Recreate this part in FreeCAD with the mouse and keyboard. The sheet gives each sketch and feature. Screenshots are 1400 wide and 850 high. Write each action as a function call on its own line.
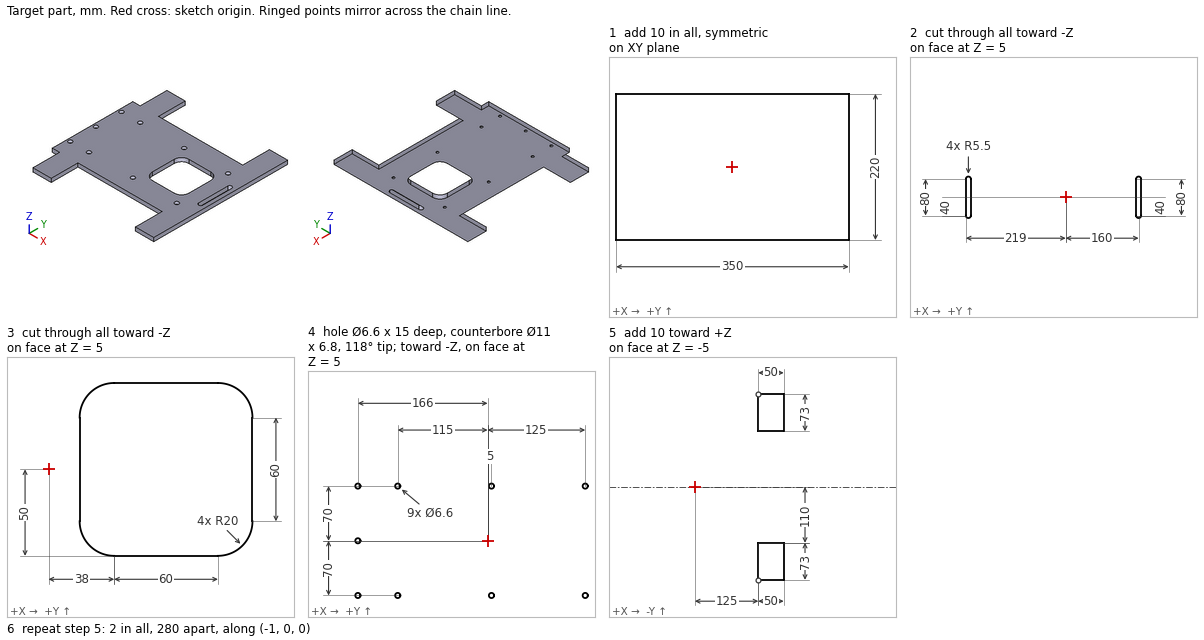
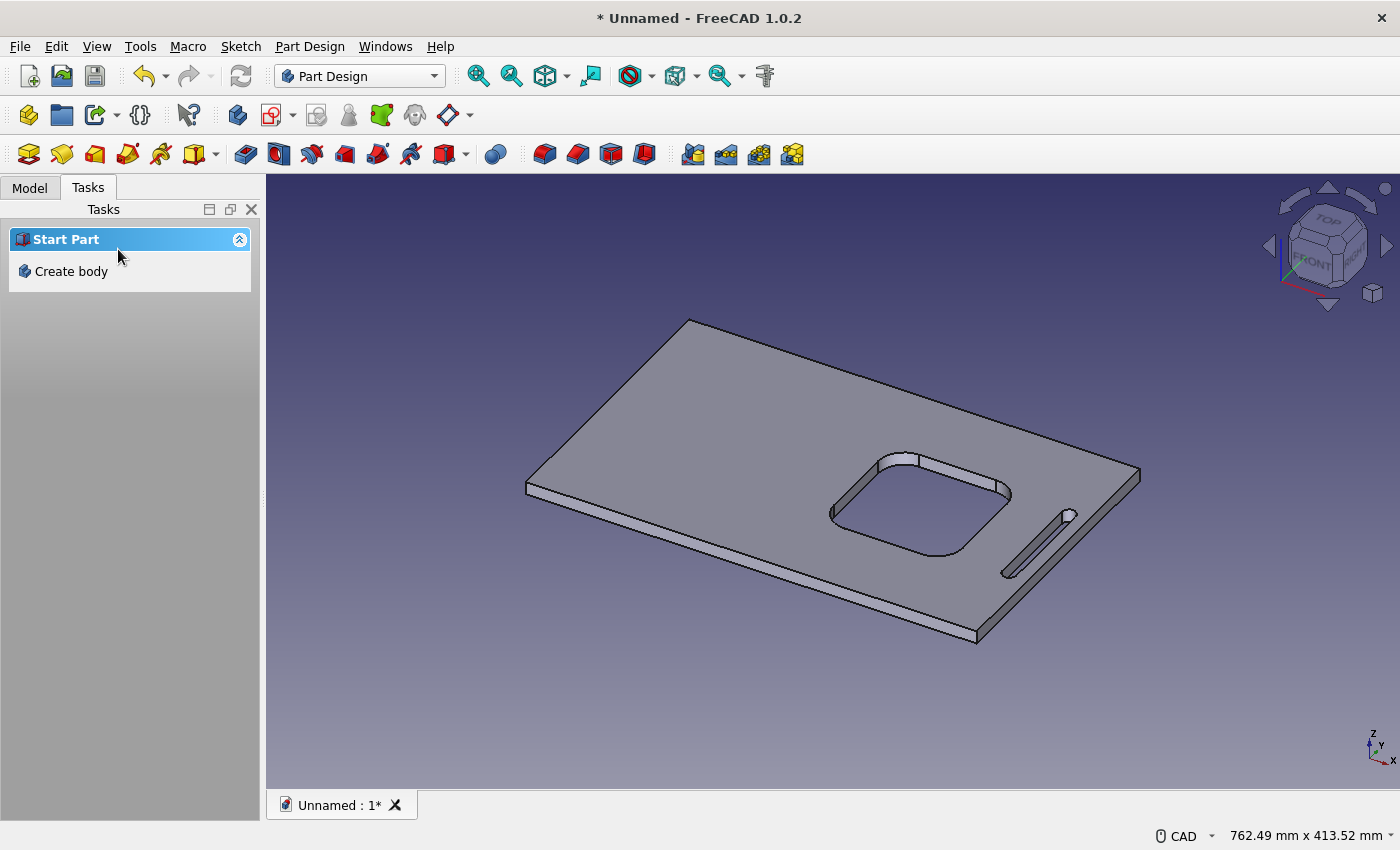
click(728, 409)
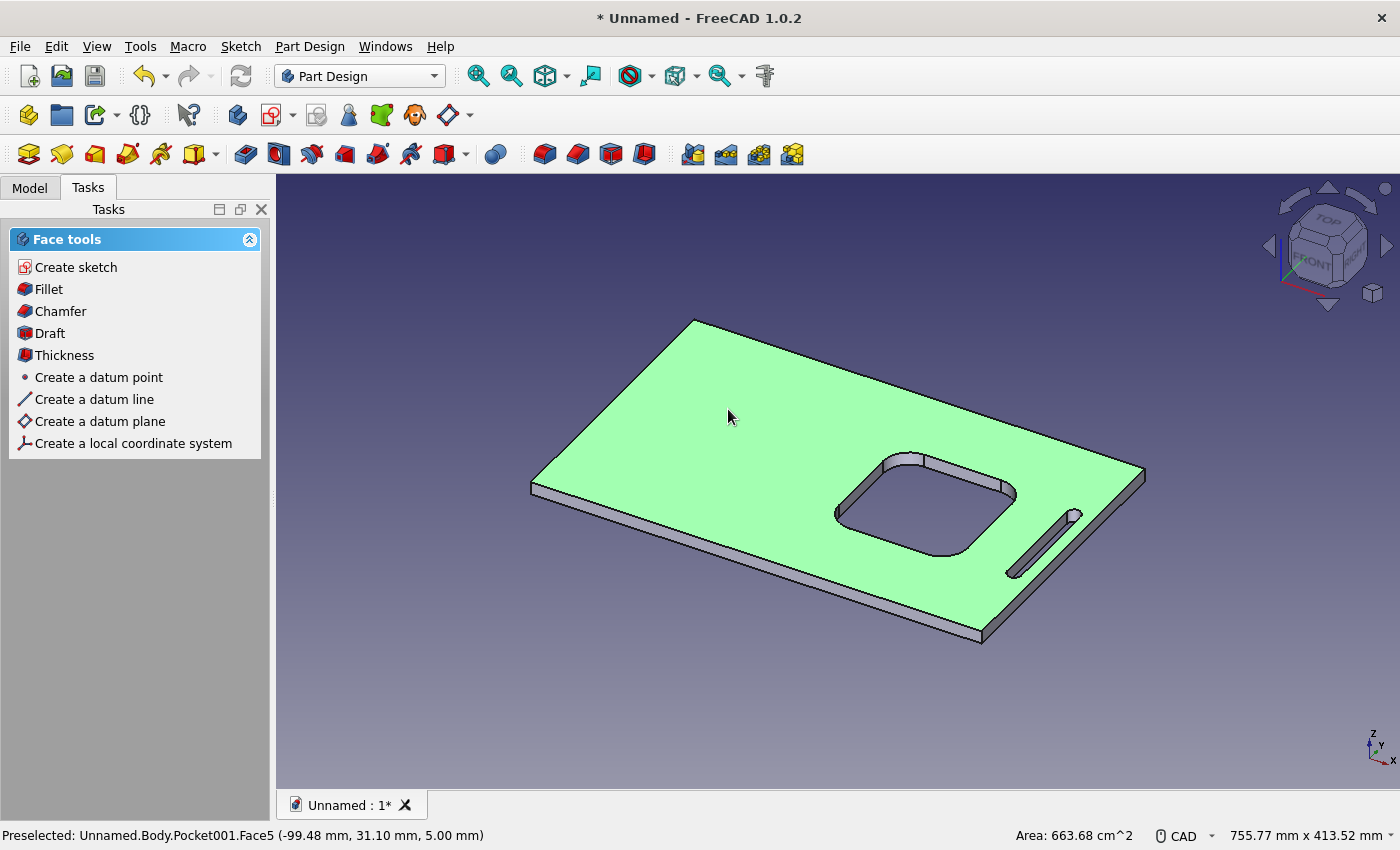
click(270, 116)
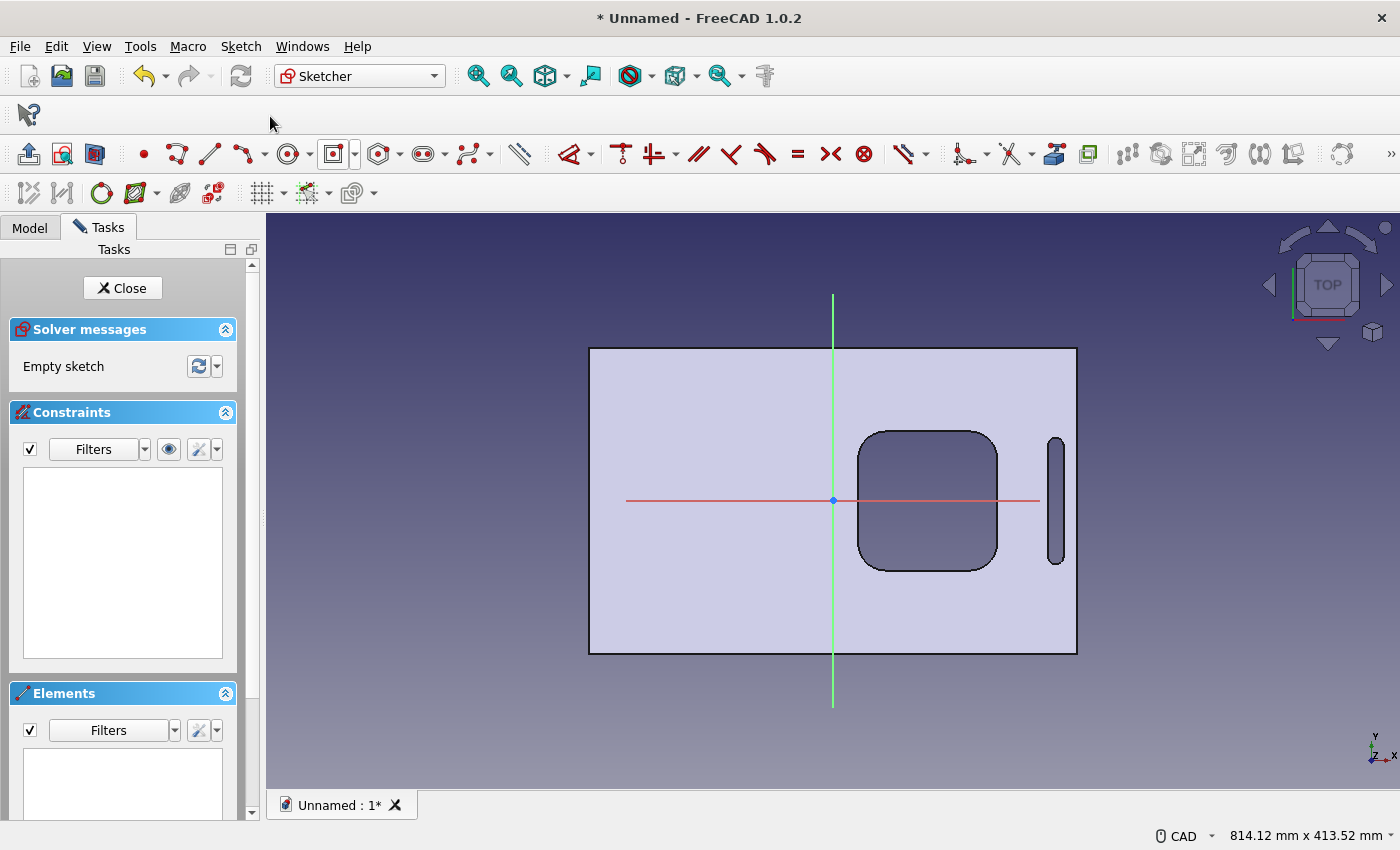
scroll(886, 501, up, 2)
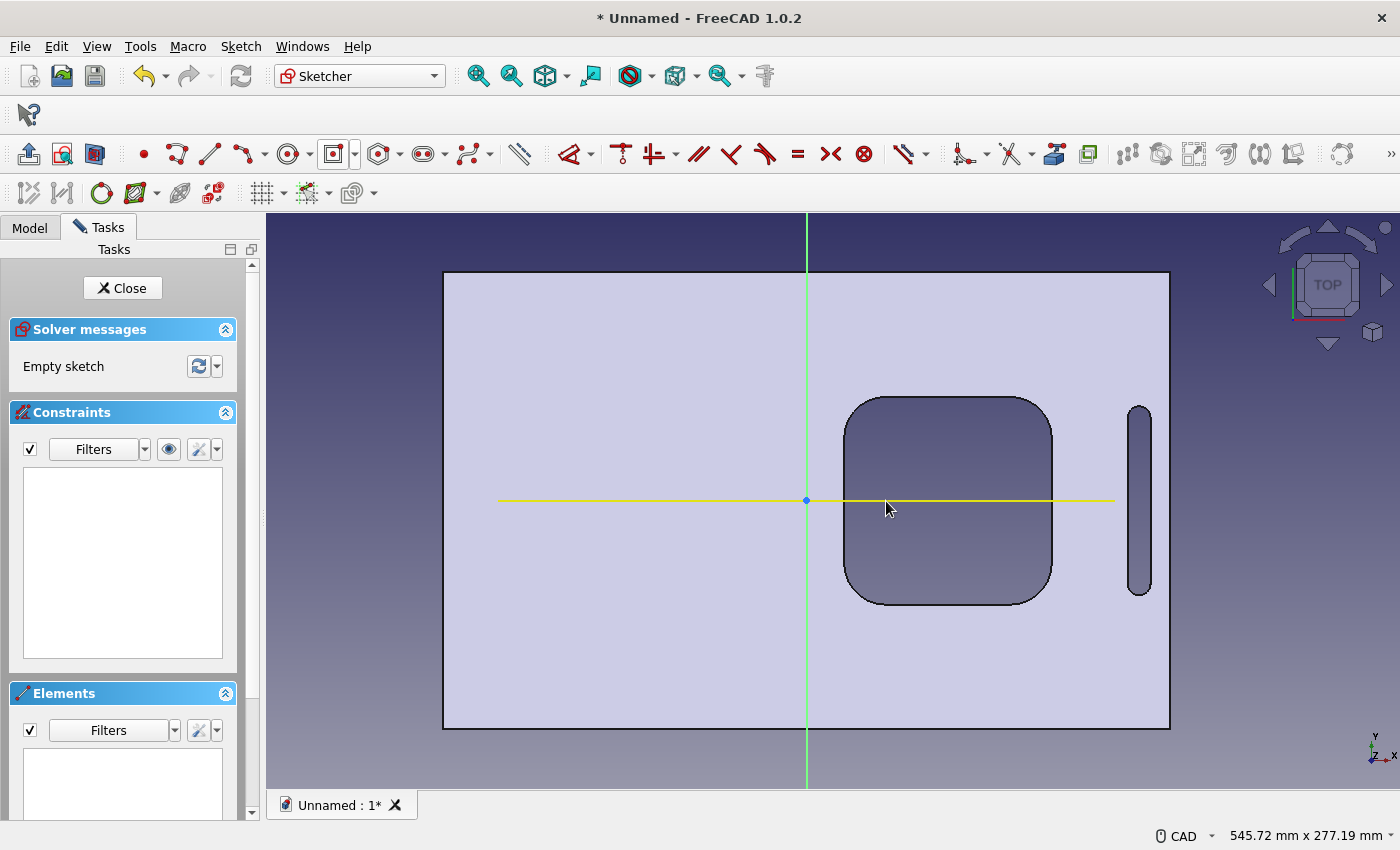
click(288, 154)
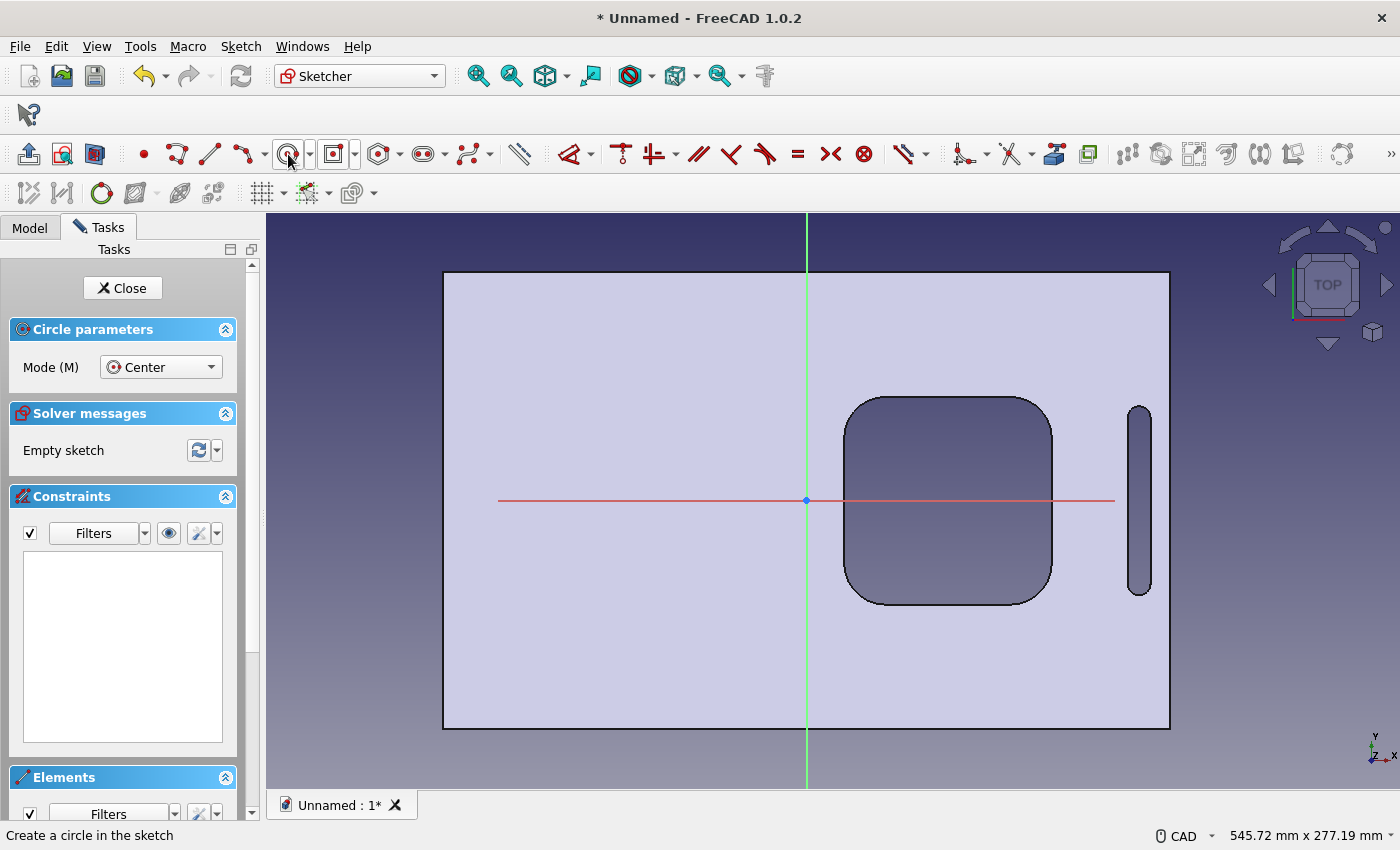
scroll(568, 355, up, 6)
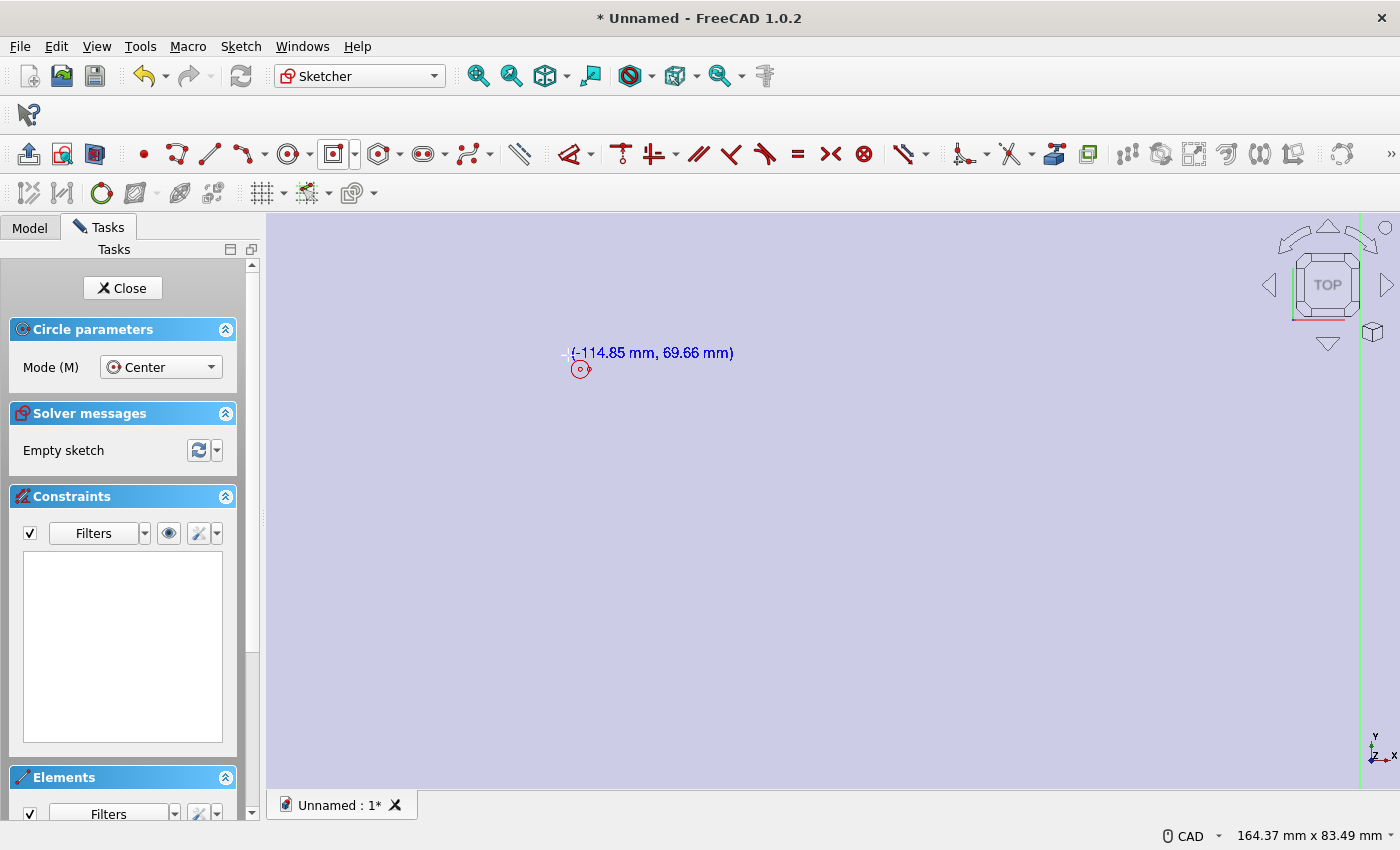
click(566, 355)
move(582, 339)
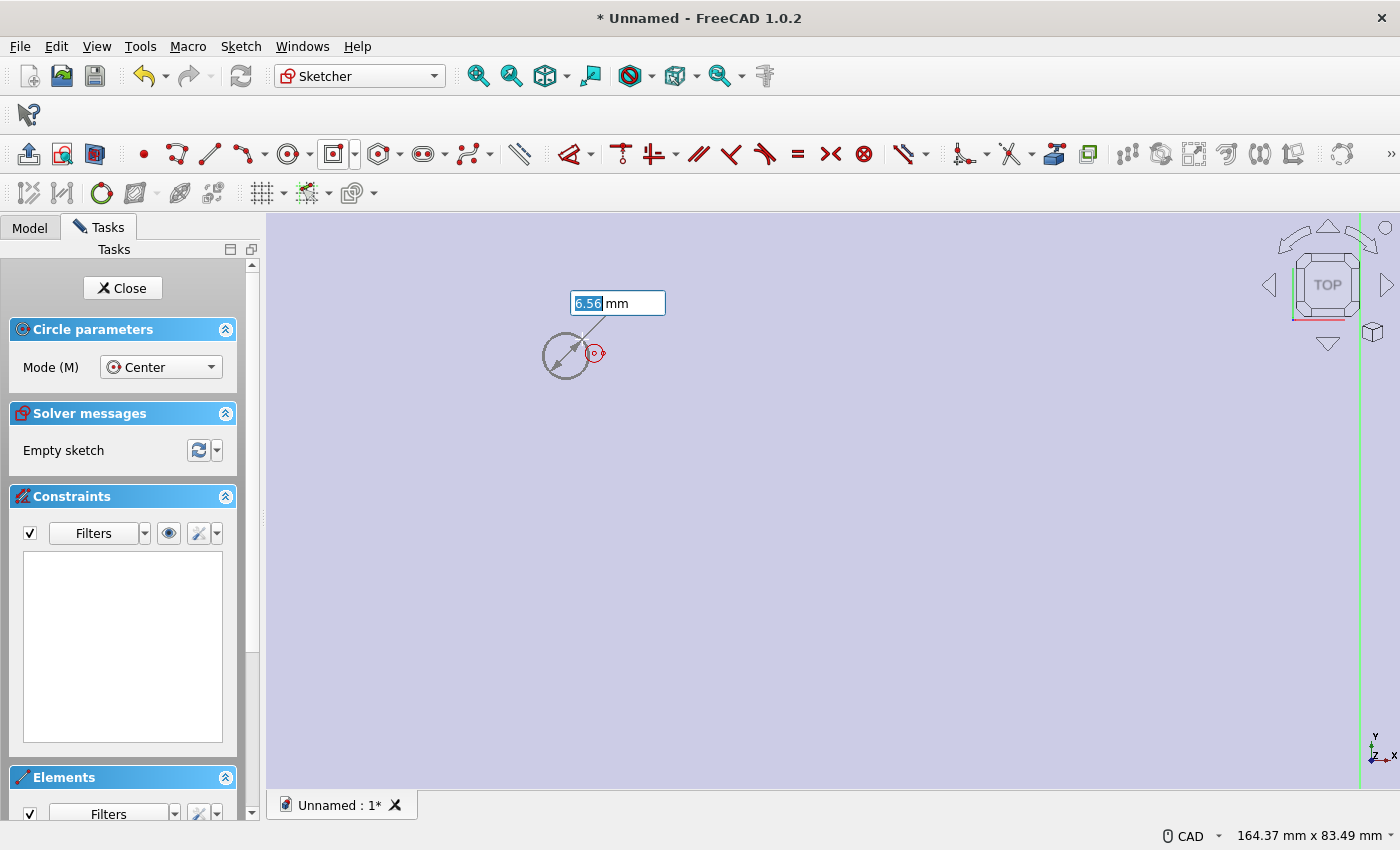
text(6.6)
key(Return)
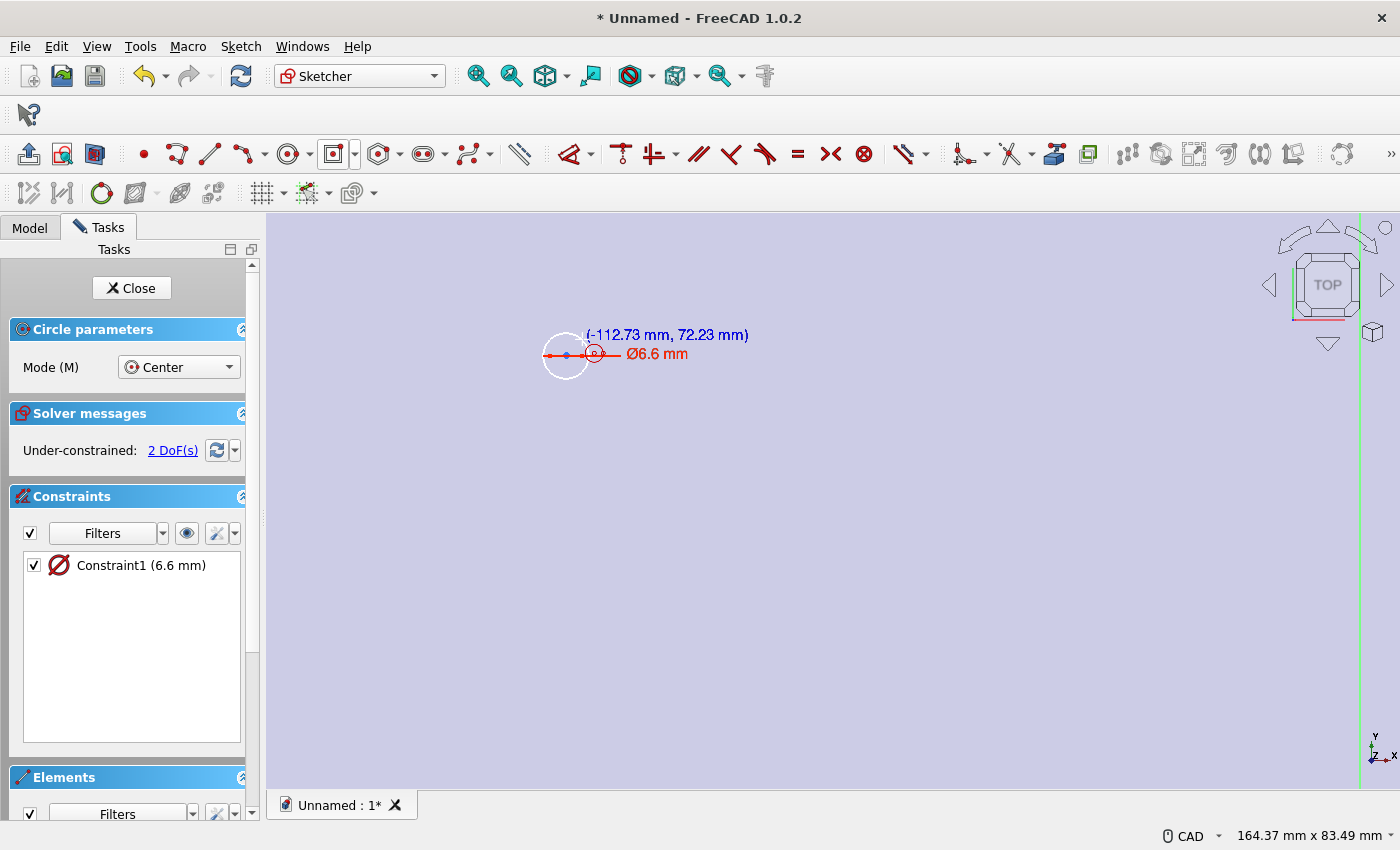
scroll(569, 356, down, 6)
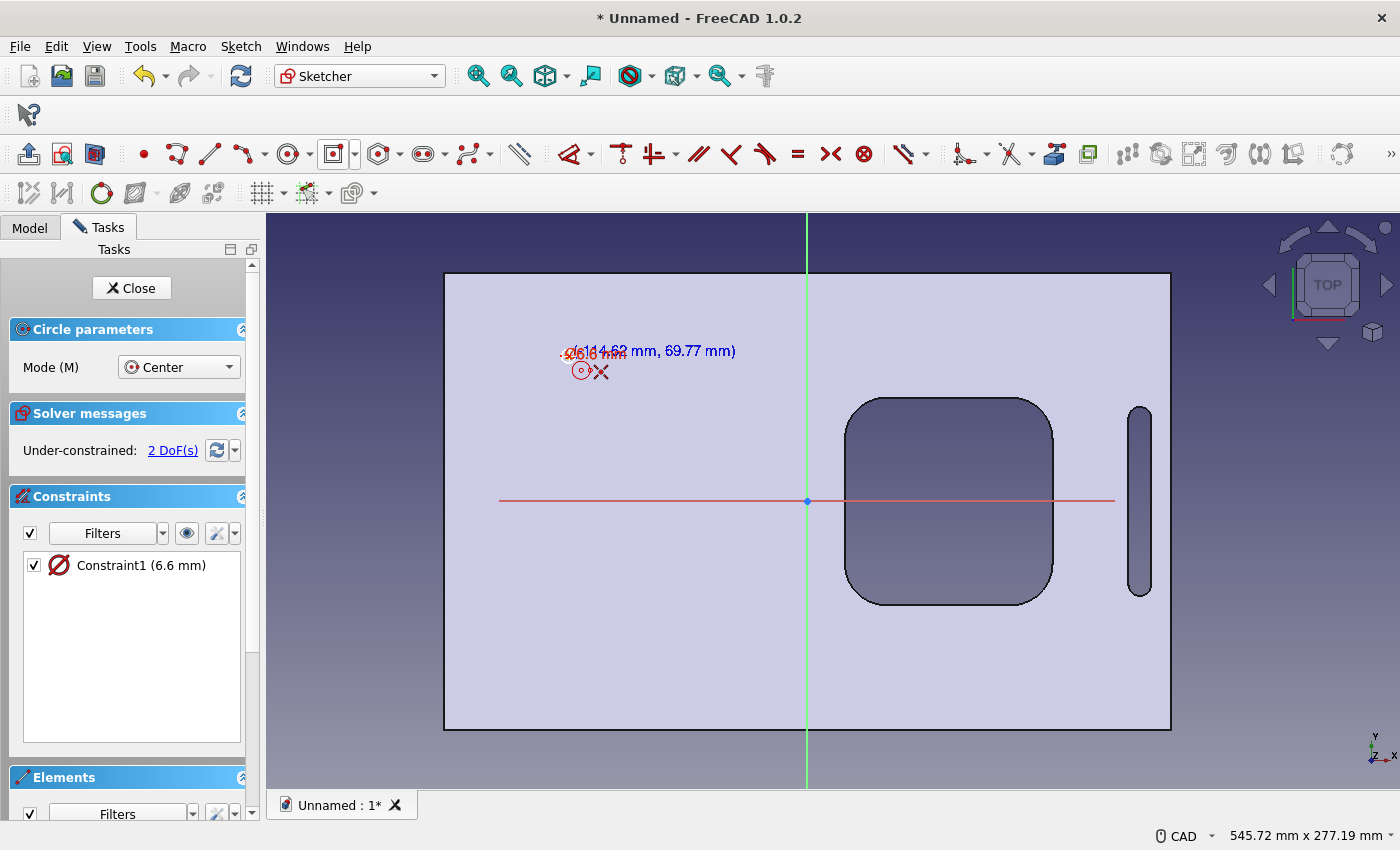
scroll(568, 647, up, 6)